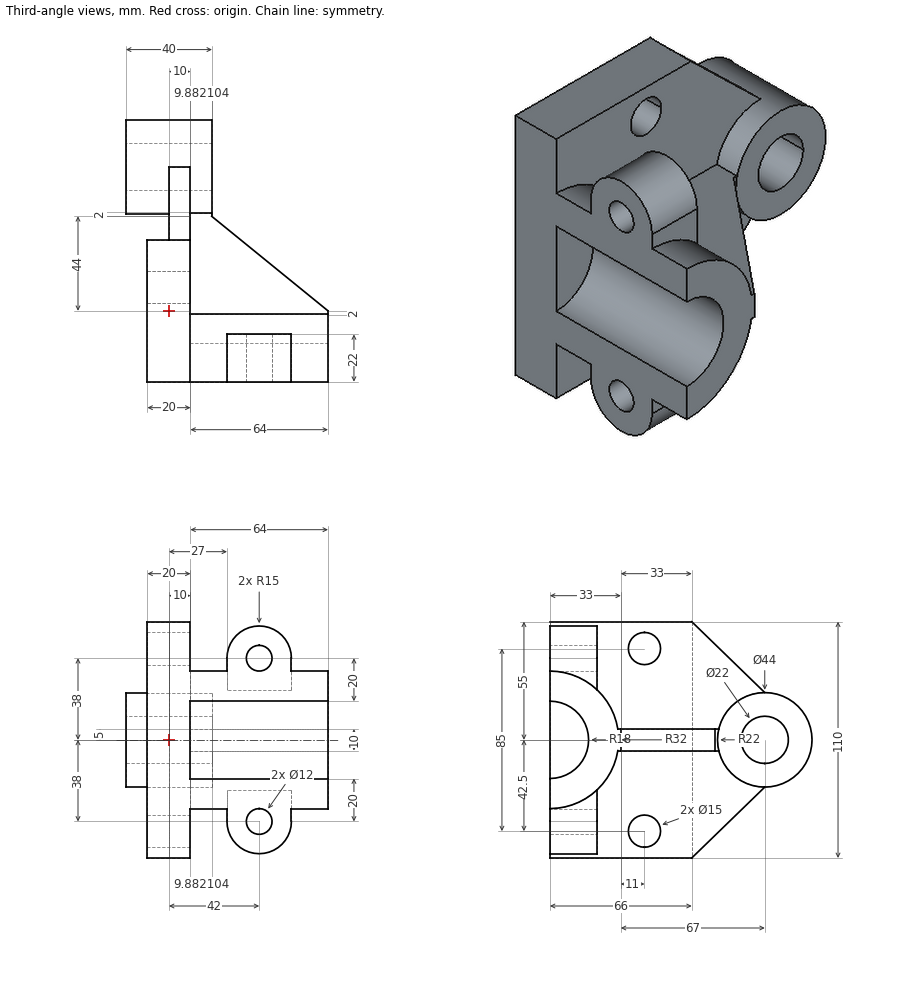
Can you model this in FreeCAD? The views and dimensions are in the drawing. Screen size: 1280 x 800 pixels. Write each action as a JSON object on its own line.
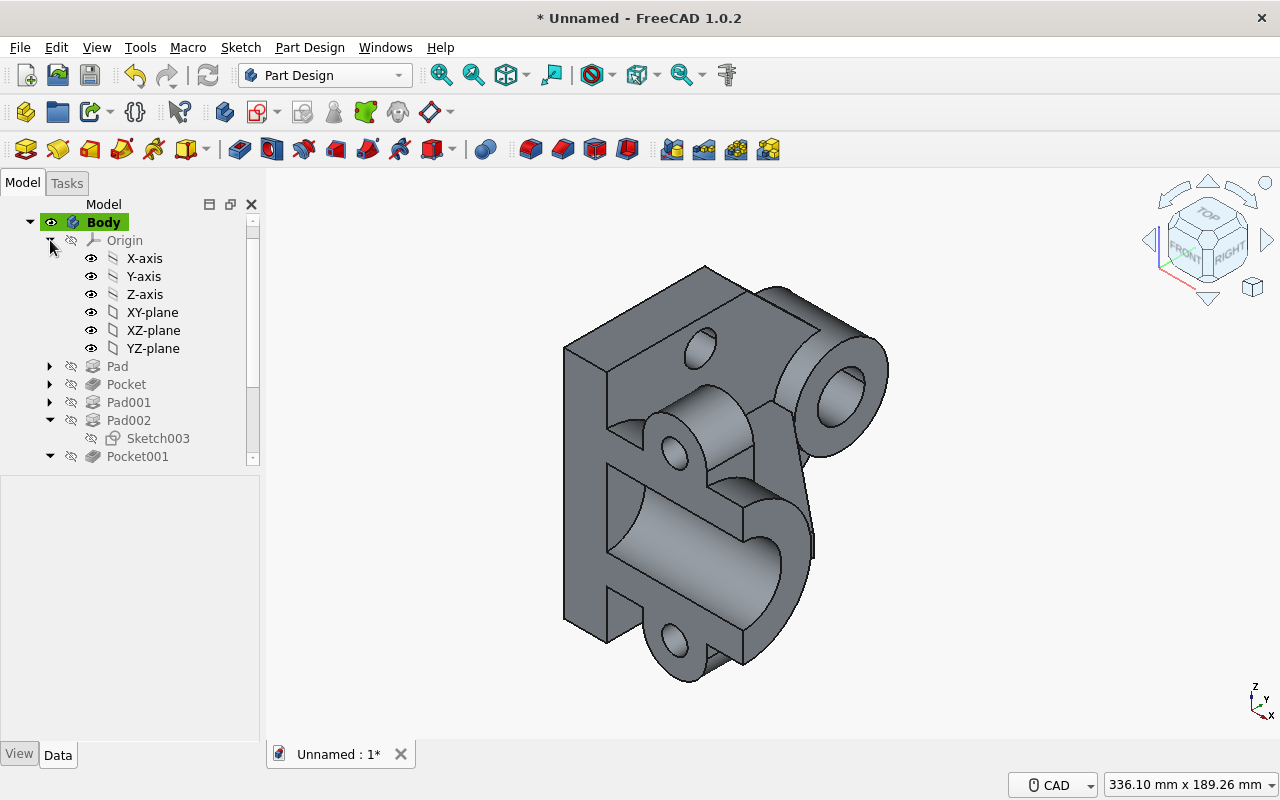
{"action": "left_click", "coordinate": [136, 330]}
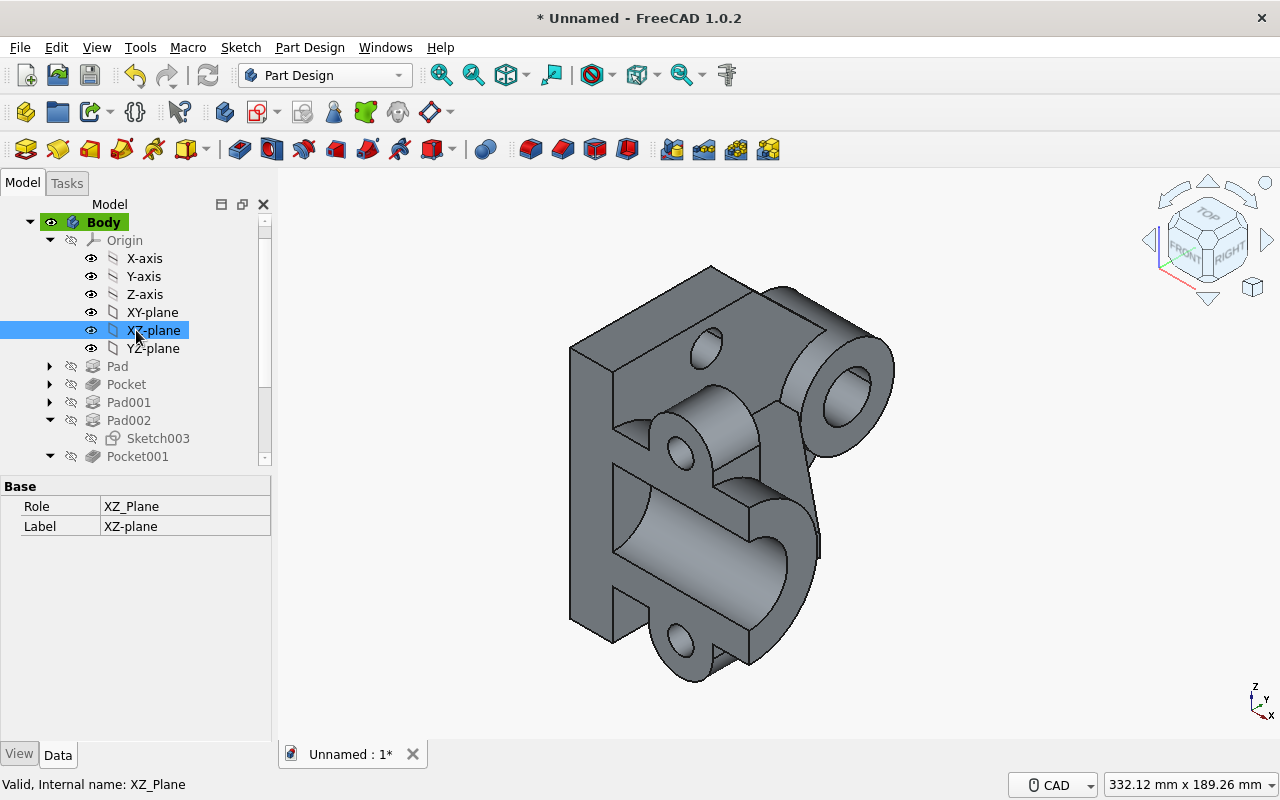
{"action": "left_click", "coordinate": [430, 112]}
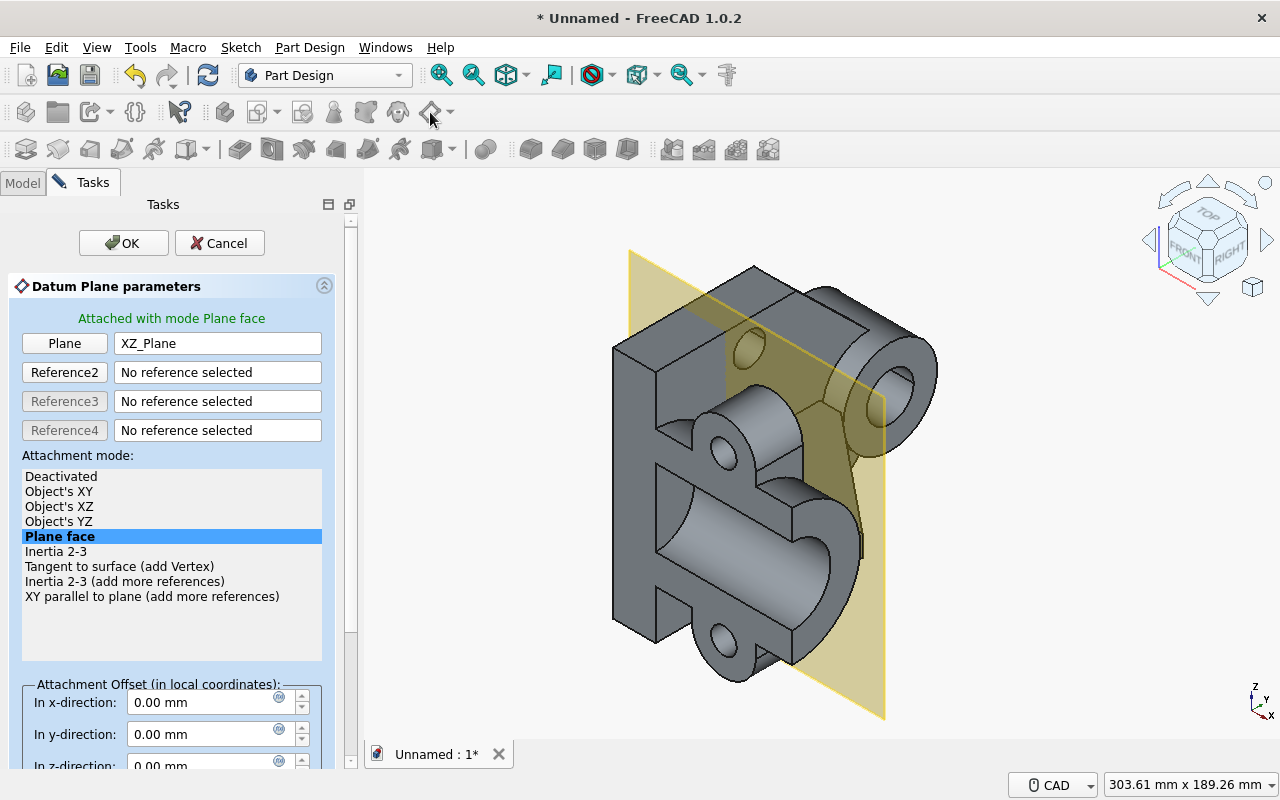
{"action": "scroll", "coordinate": [351, 491], "scroll_direction": "down", "scroll_amount": 2}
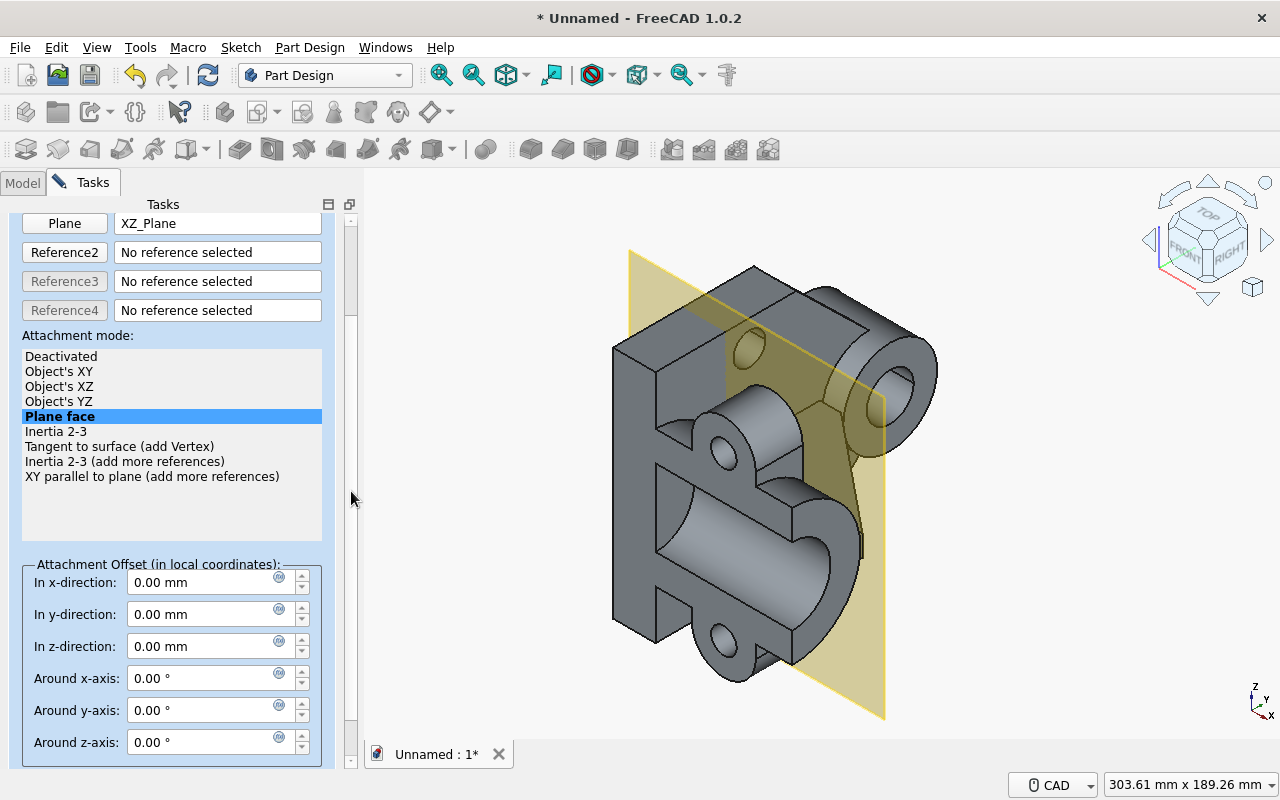
{"action": "triple_click", "coordinate": [210, 646]}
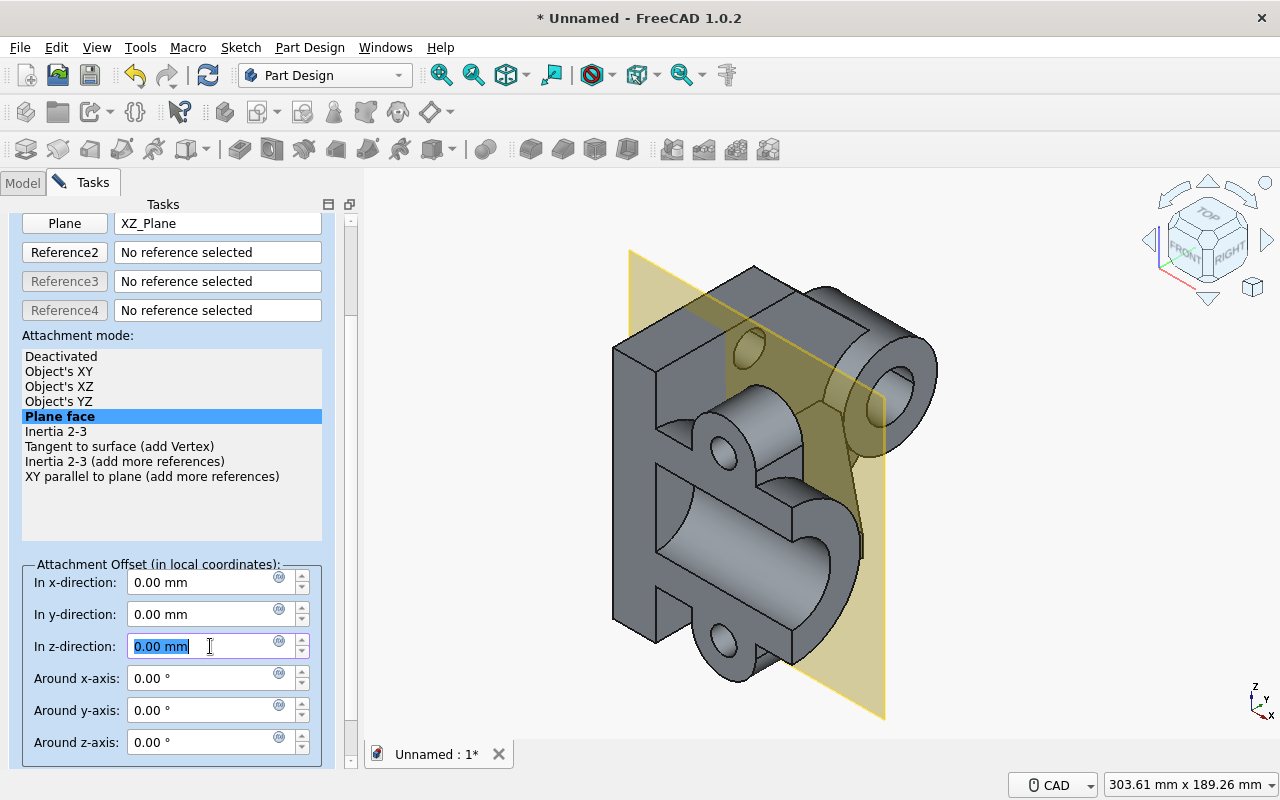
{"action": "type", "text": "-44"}
{"action": "key", "text": "Tab"}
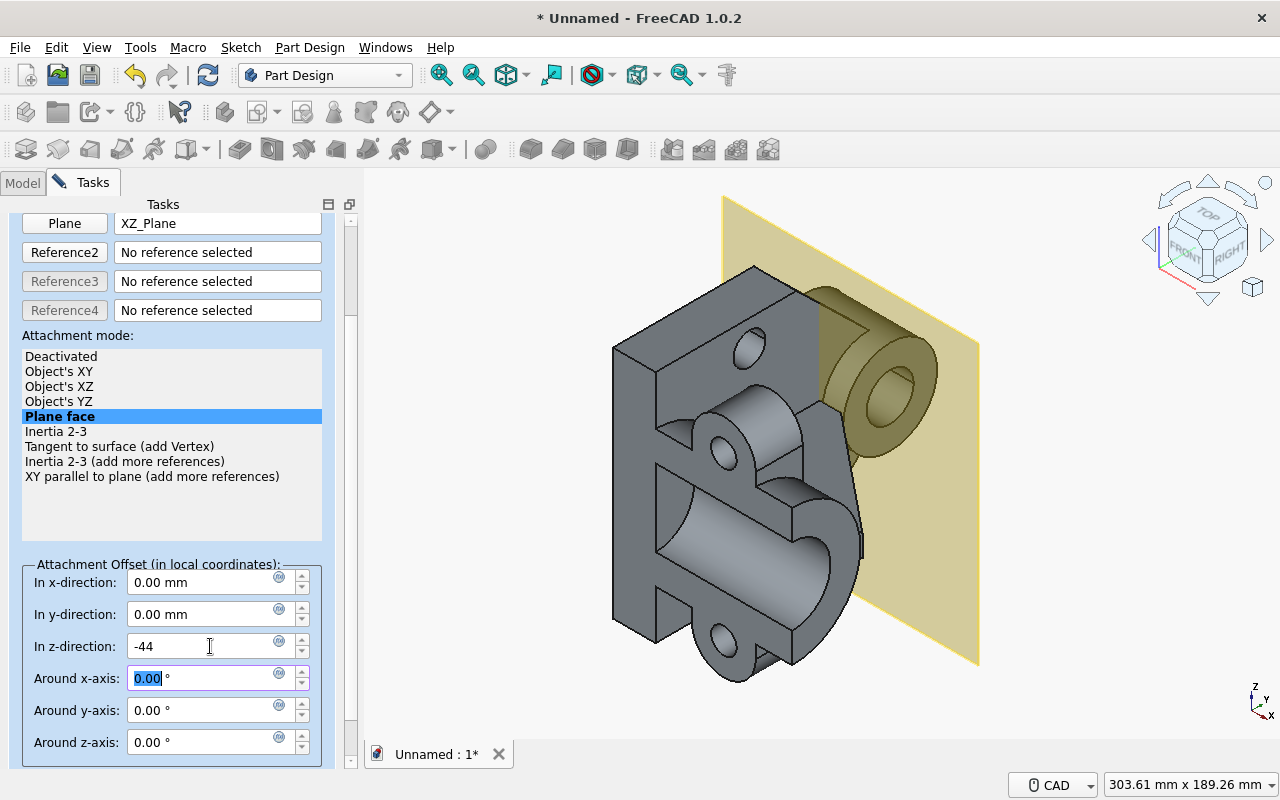
{"action": "scroll", "coordinate": [351, 491], "scroll_direction": "up", "scroll_amount": 3}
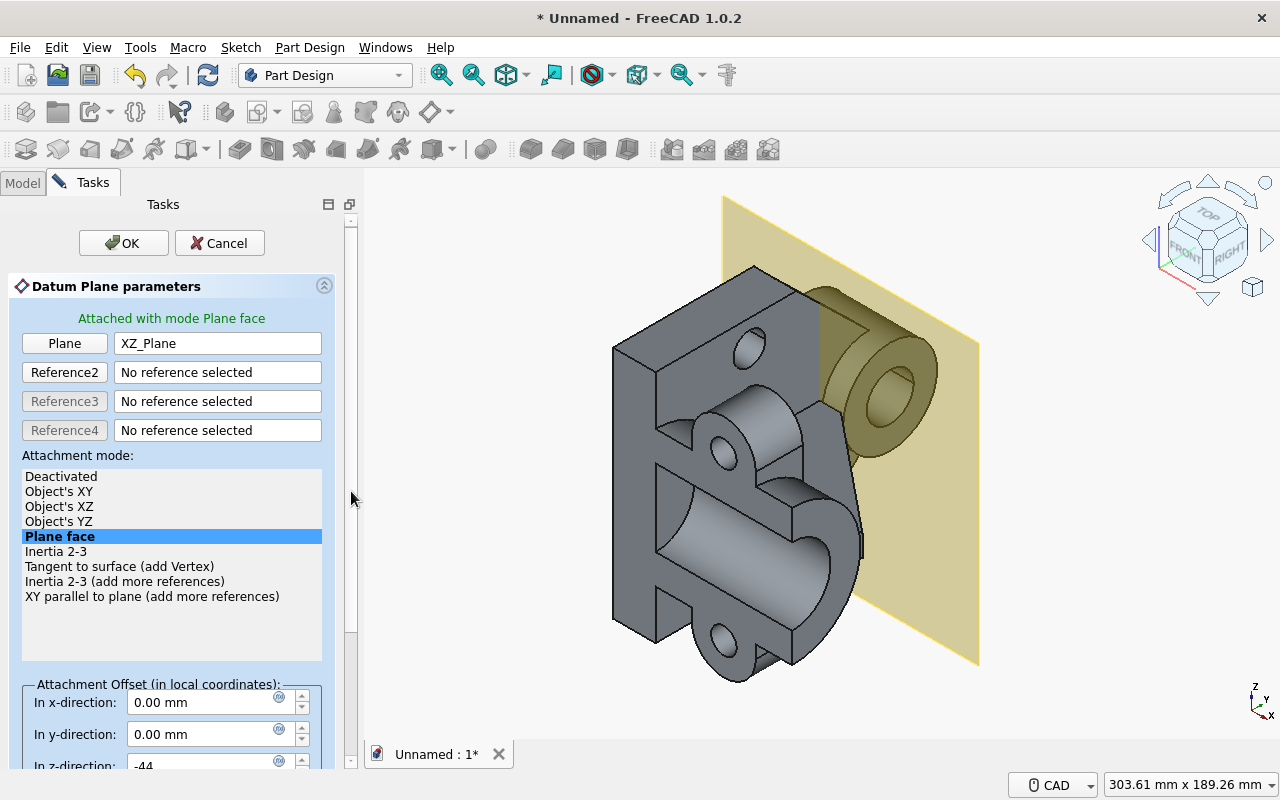
{"action": "left_click", "coordinate": [124, 243]}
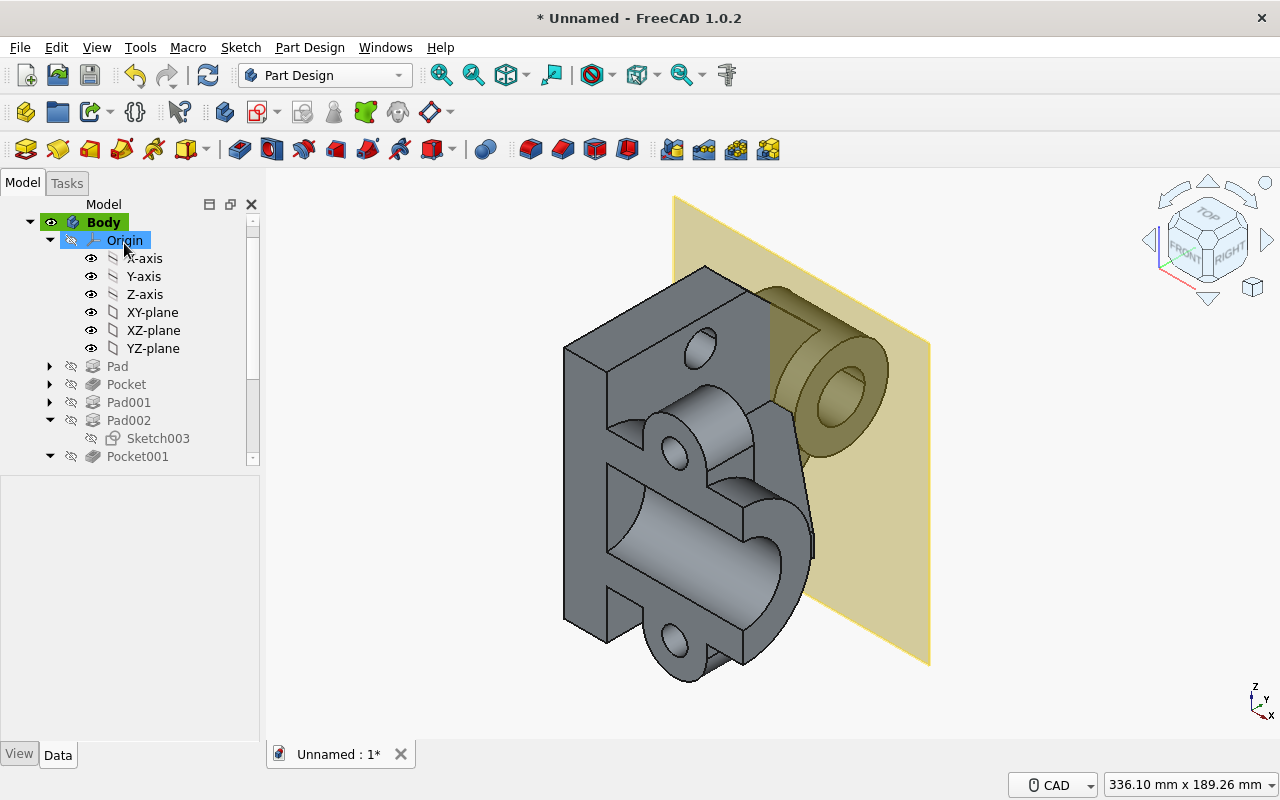
{"action": "scroll", "coordinate": [120, 344], "scroll_direction": "down", "scroll_amount": 3}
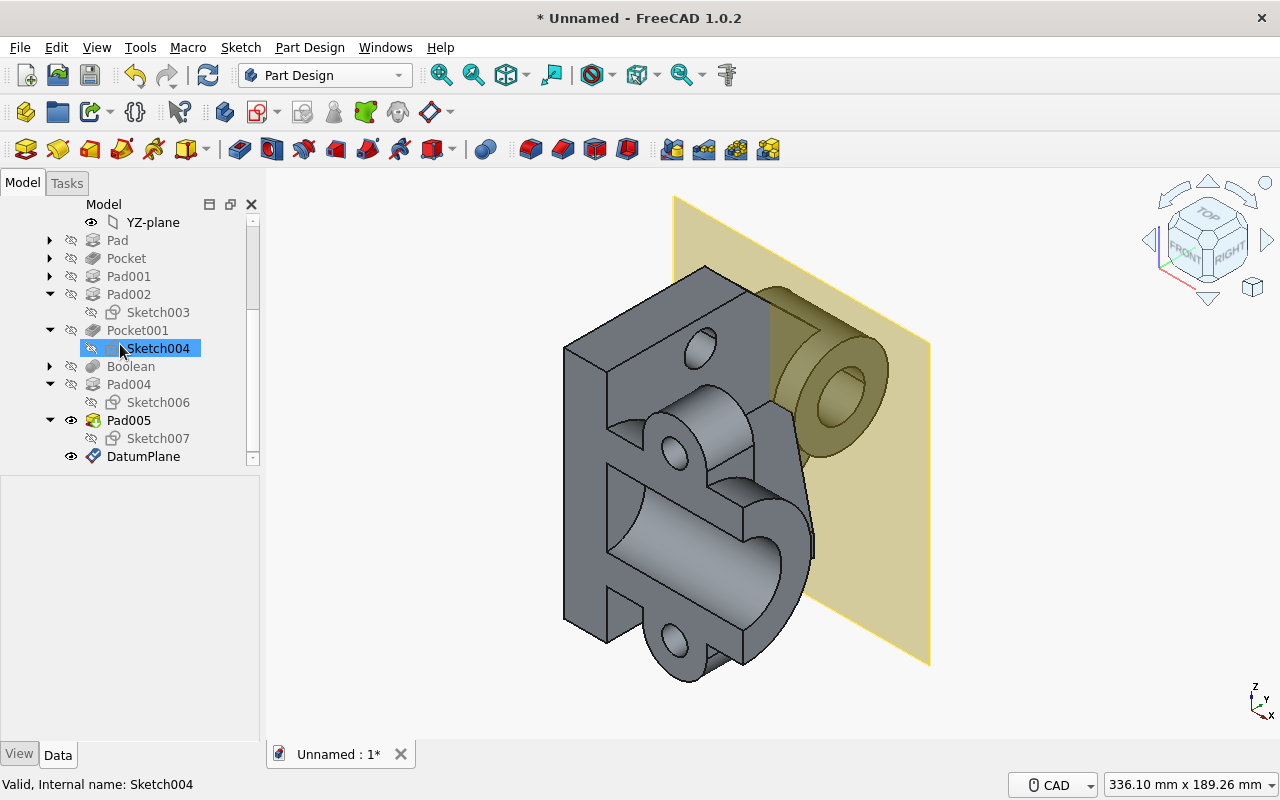
{"action": "left_click", "coordinate": [116, 456]}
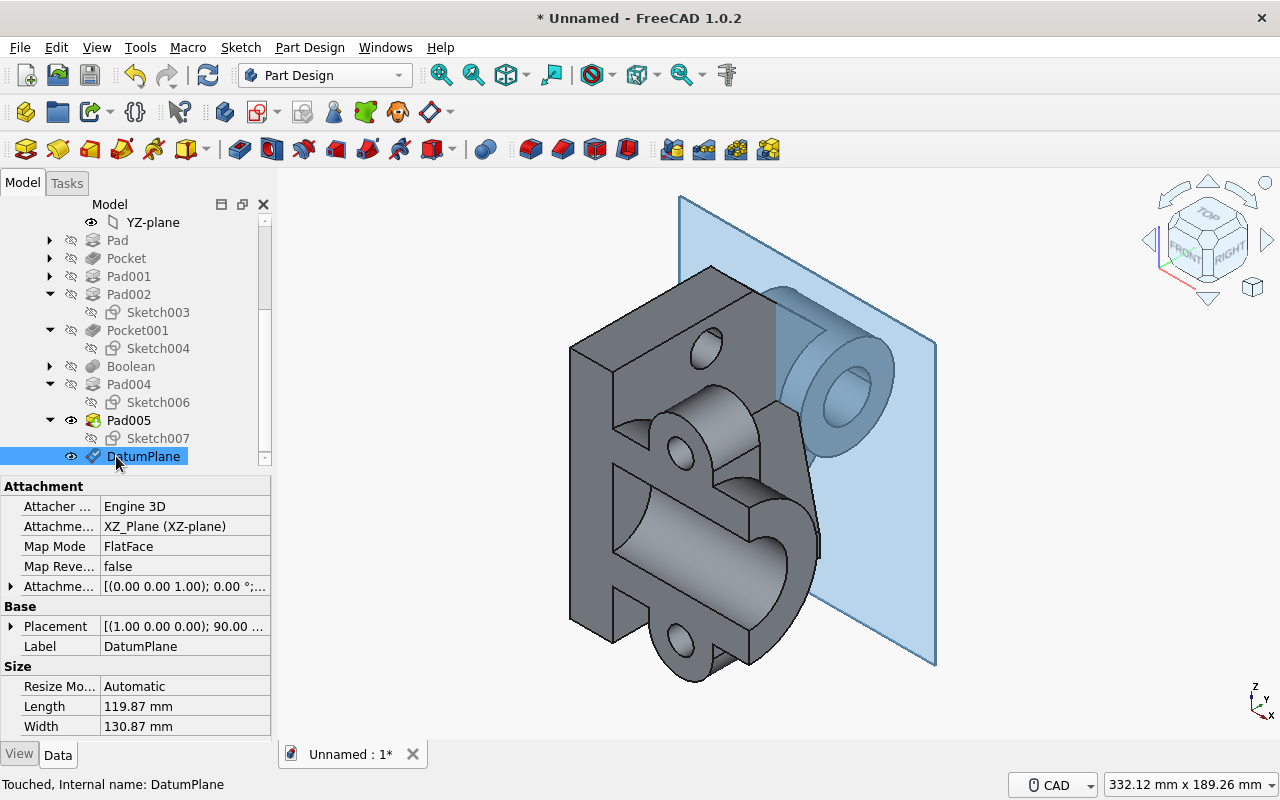
{"action": "left_click", "coordinate": [258, 112]}